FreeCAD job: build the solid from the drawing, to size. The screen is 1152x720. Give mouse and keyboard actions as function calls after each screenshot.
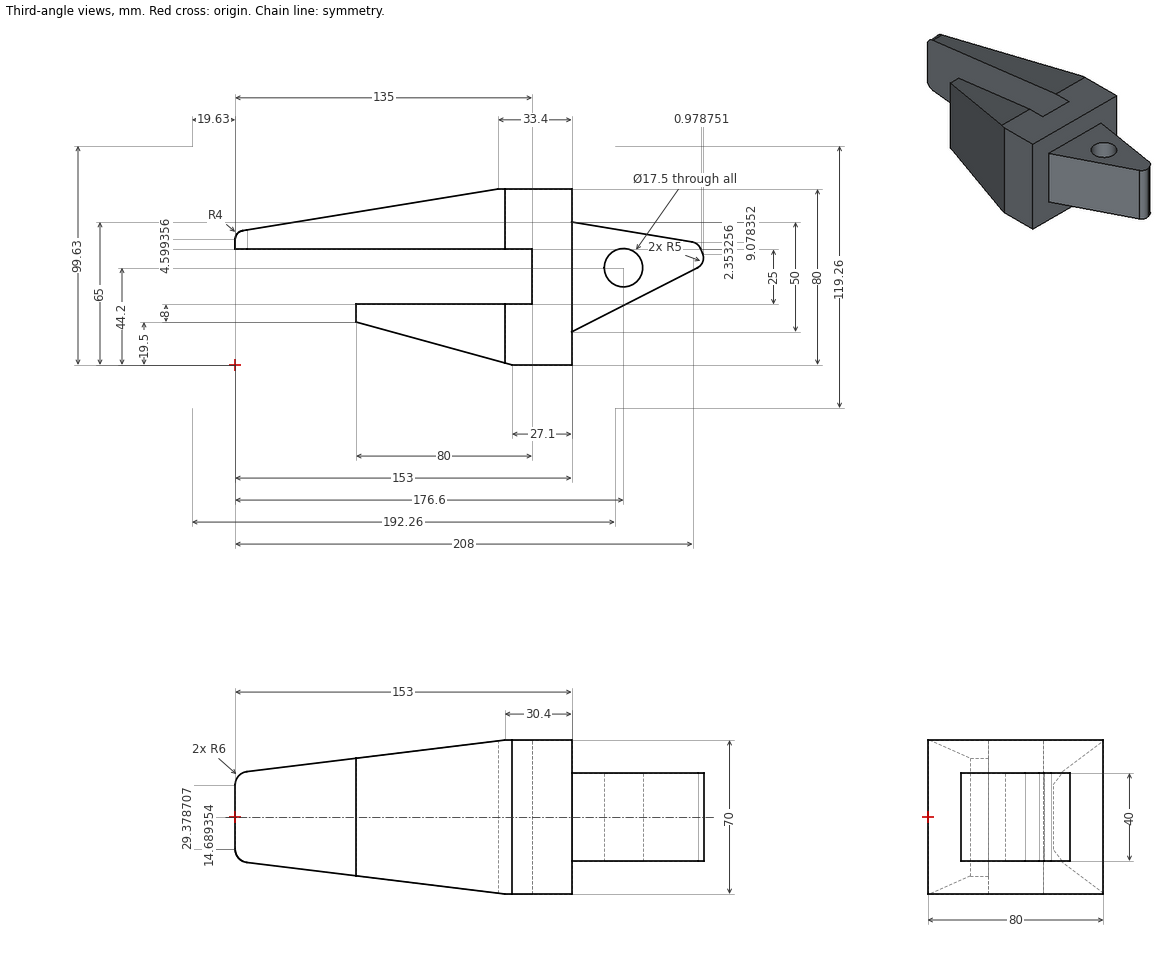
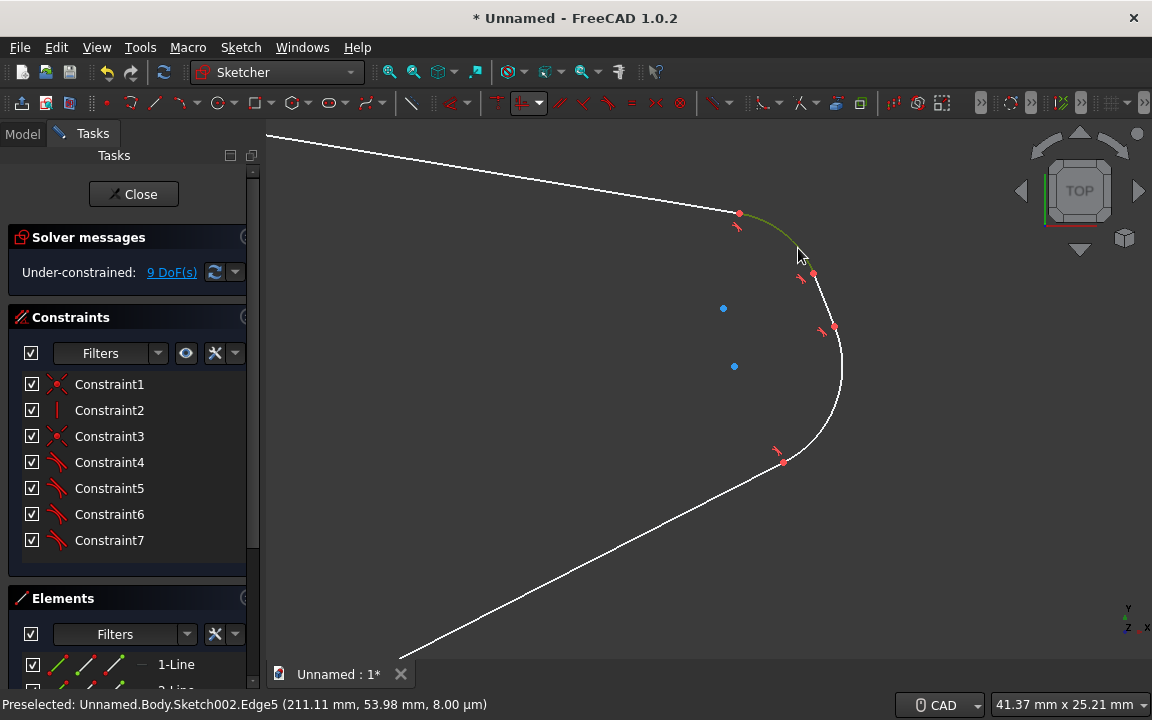
click(820, 432)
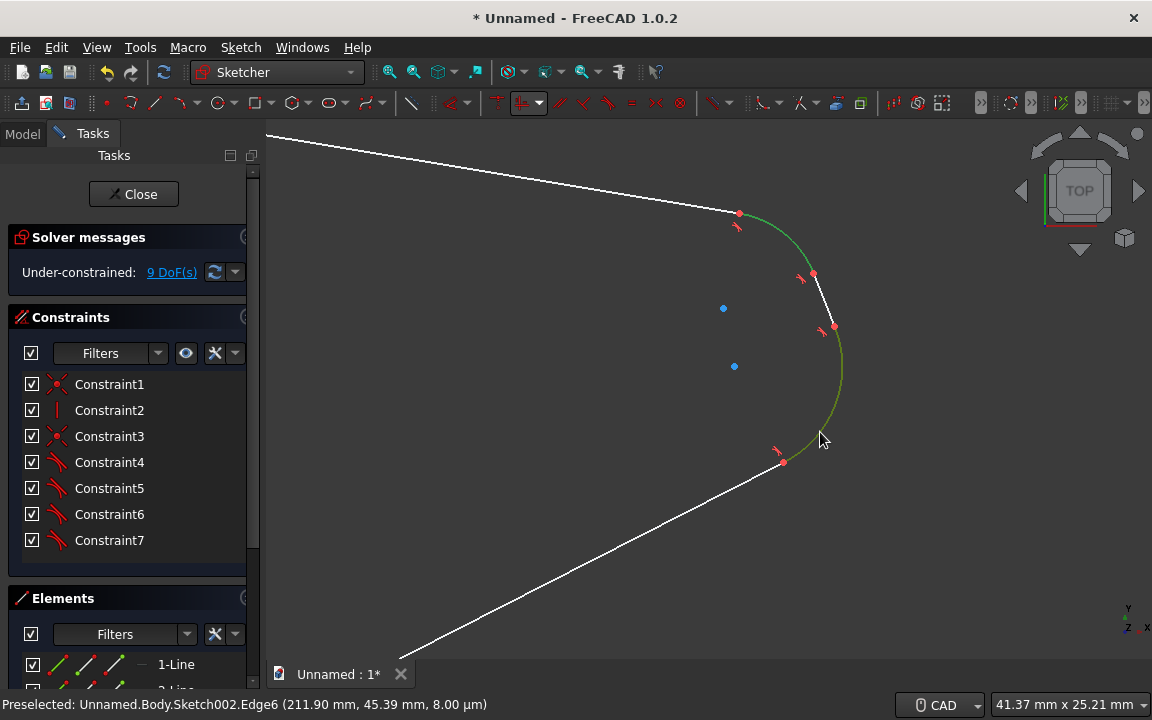
click(632, 104)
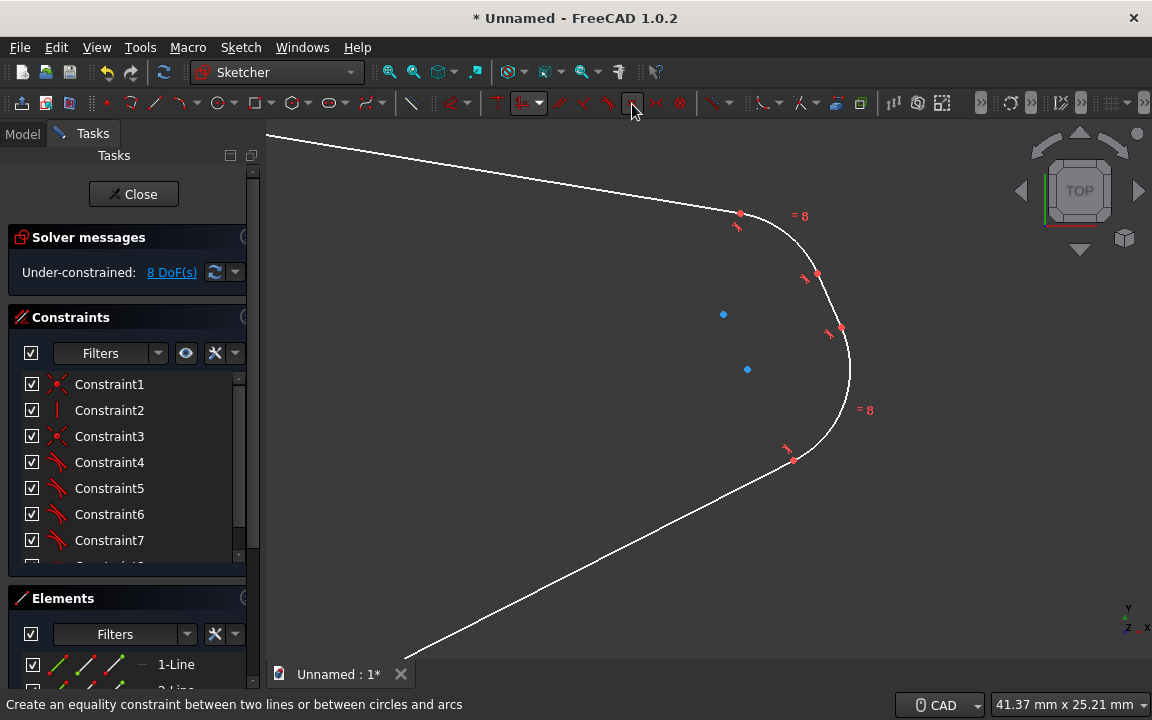
key(d)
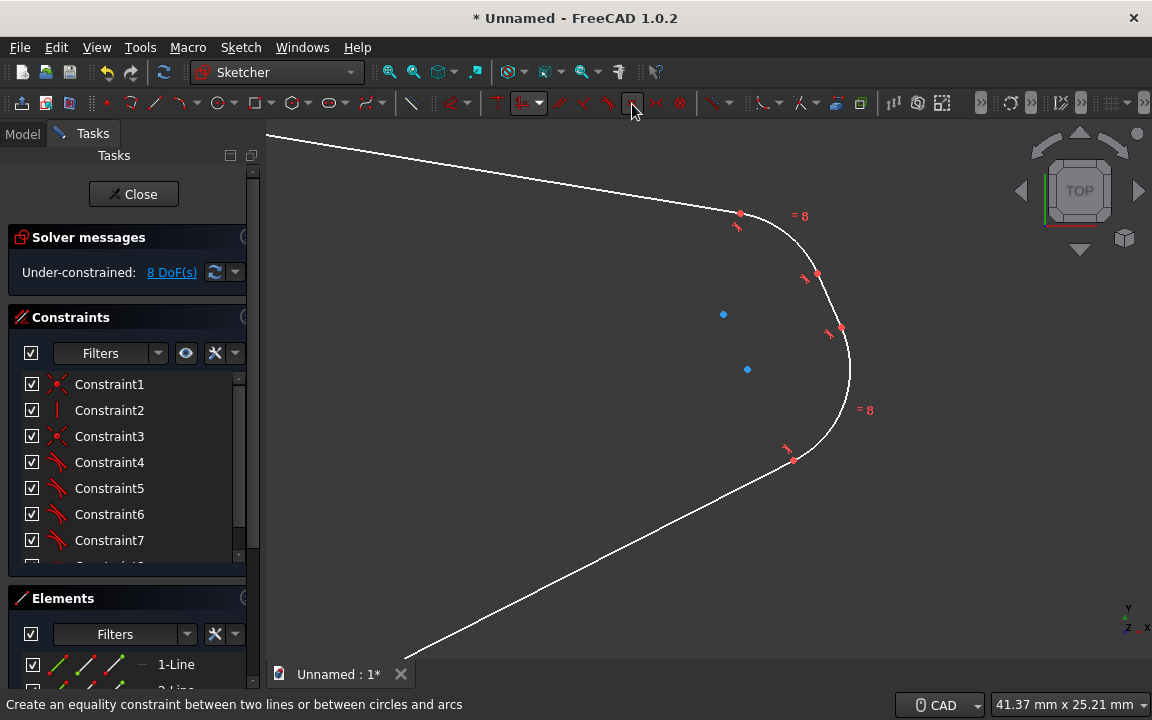
click(801, 247)
click(825, 226)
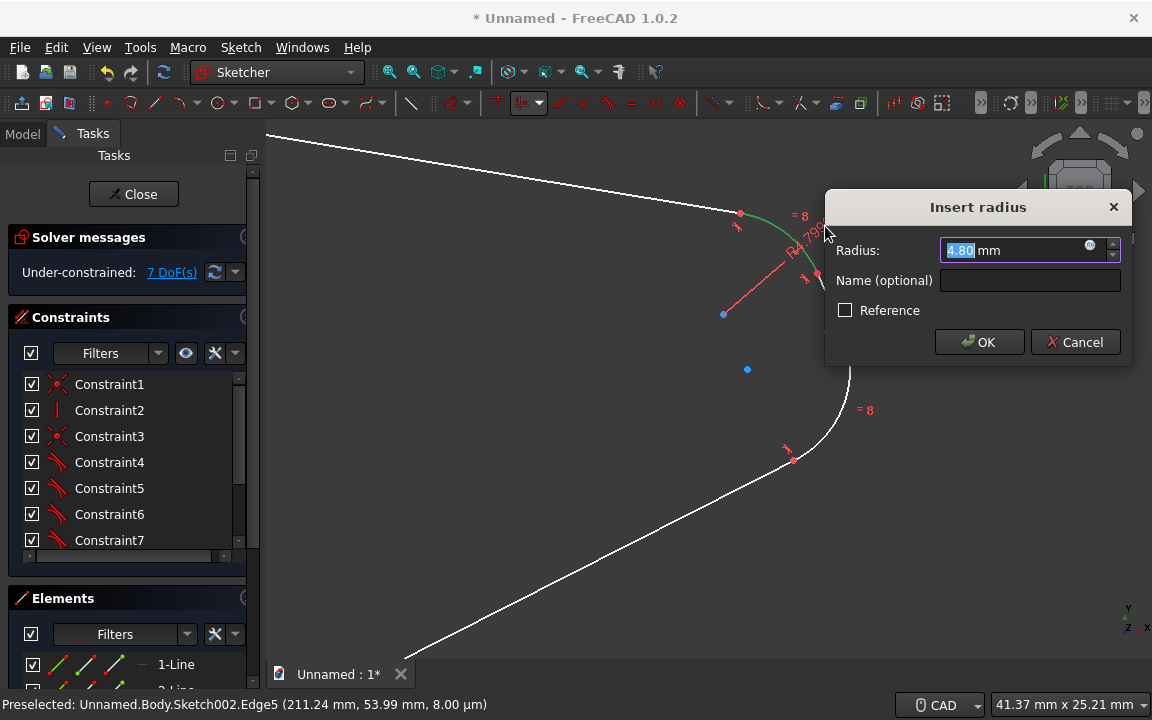
text(5)
key(Return)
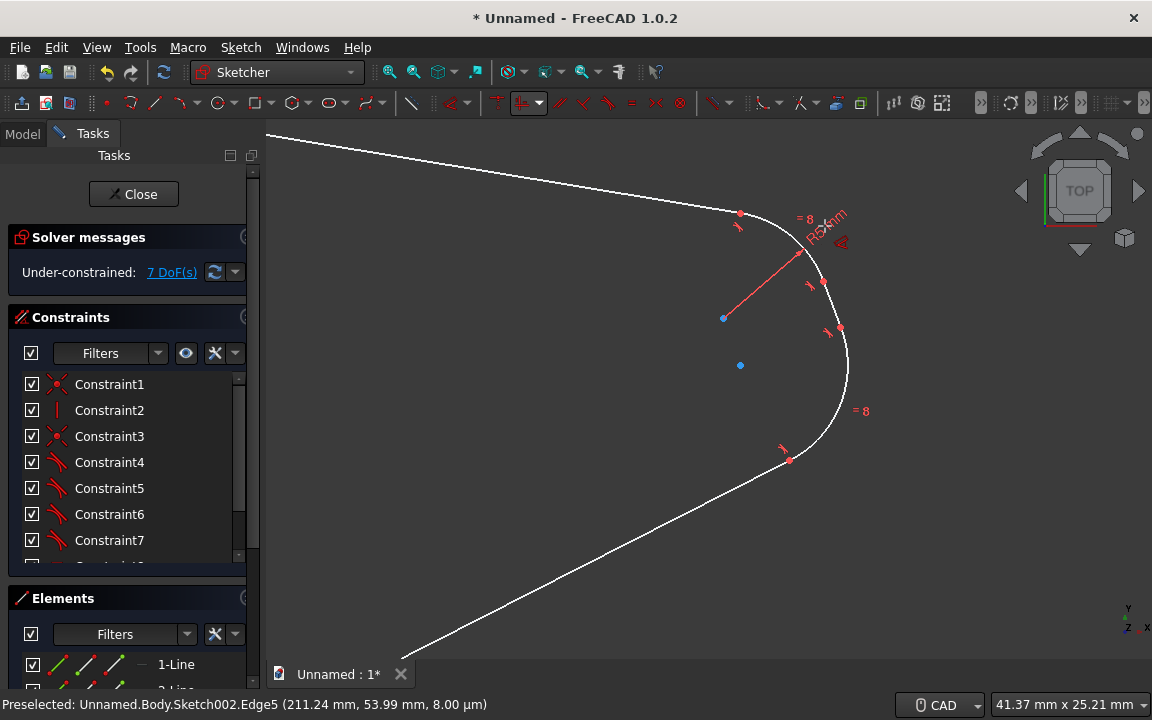
scroll(832, 319, down, 6)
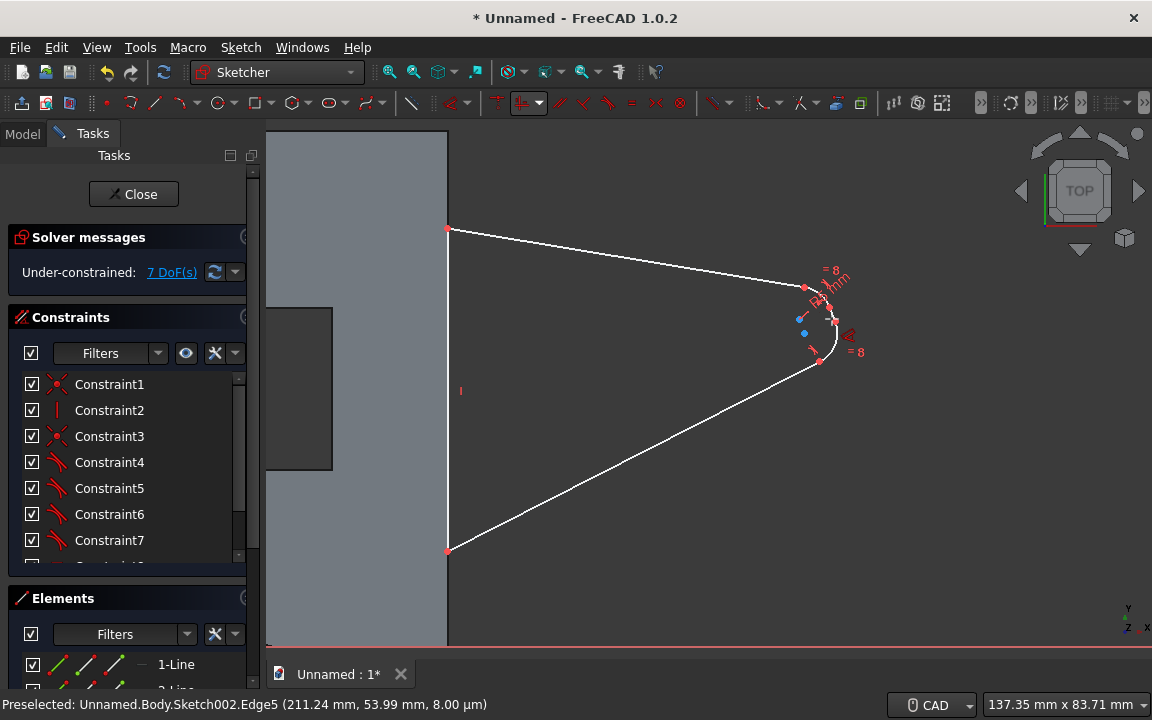
click(448, 325)
click(414, 390)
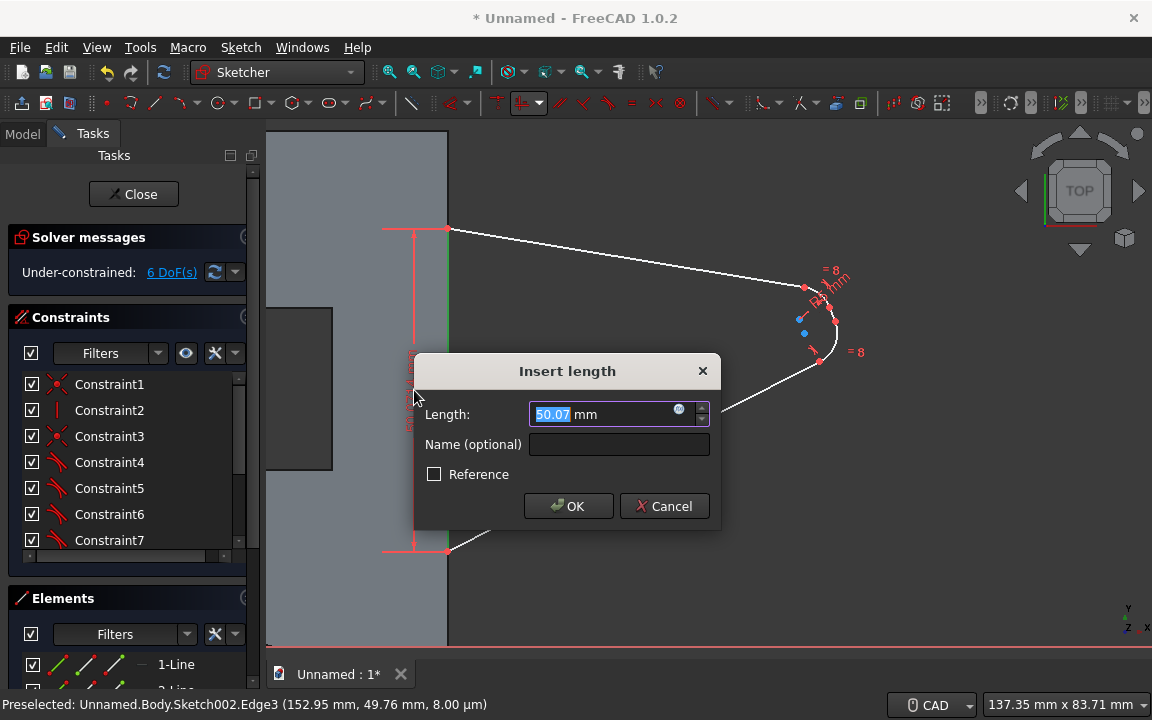
text(50)
key(Return)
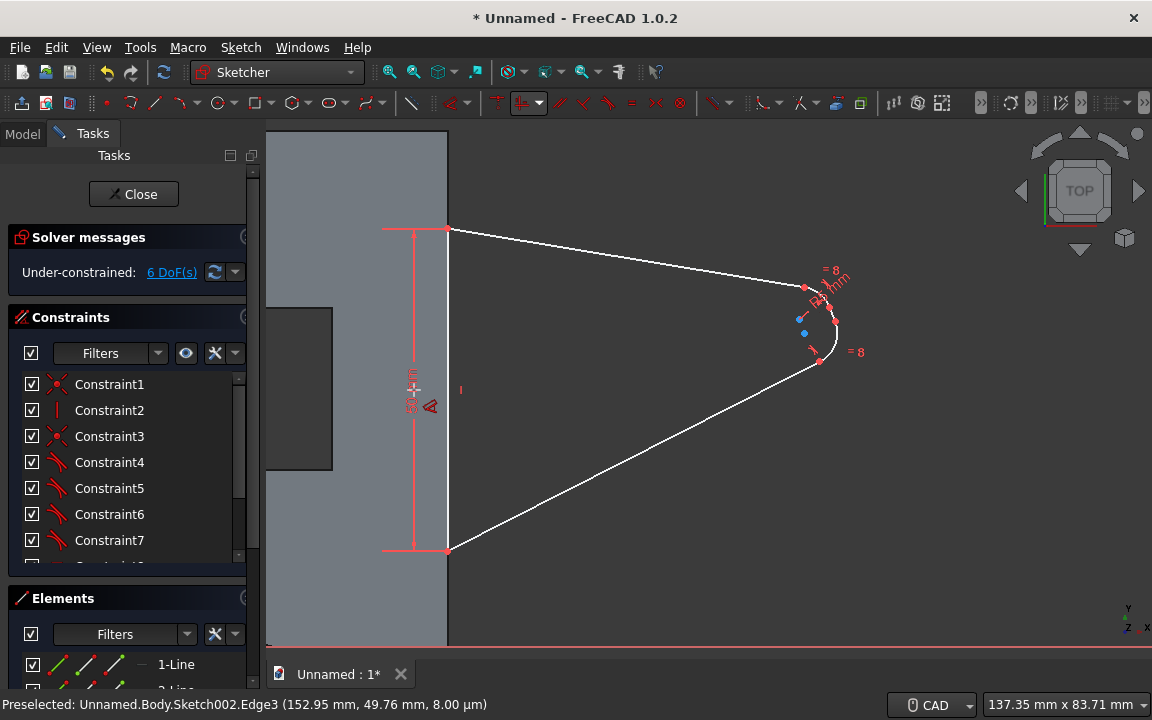
click(448, 229)
click(482, 430)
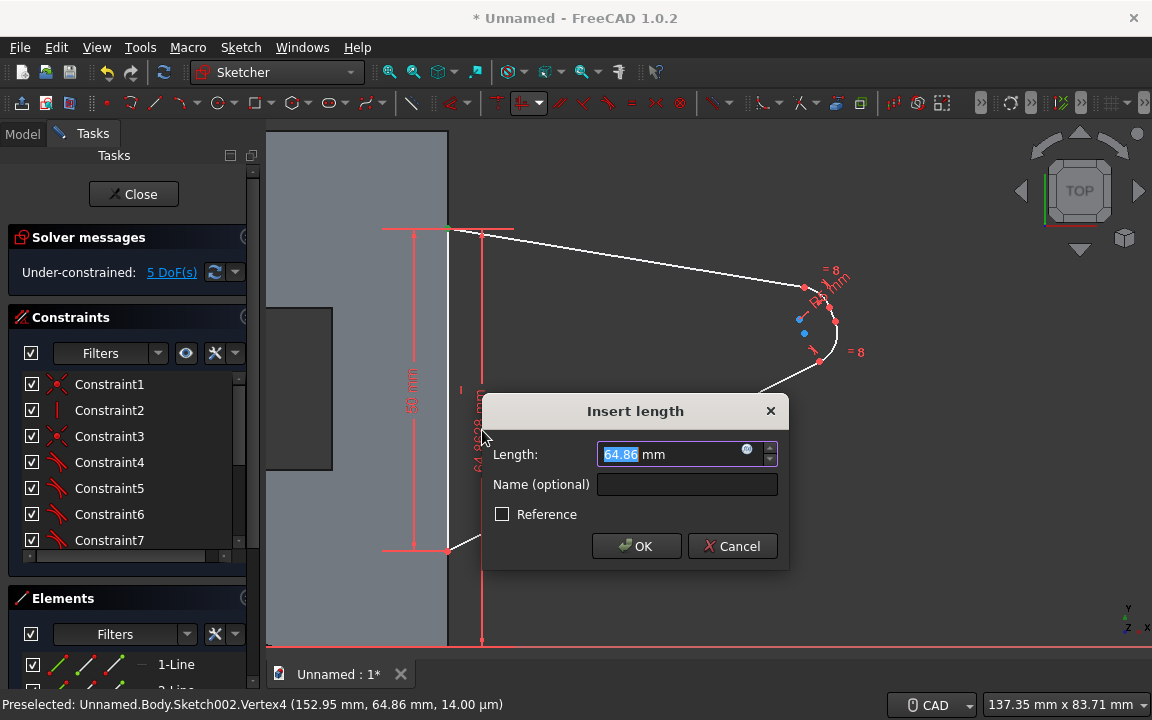
text(65)
key(Return)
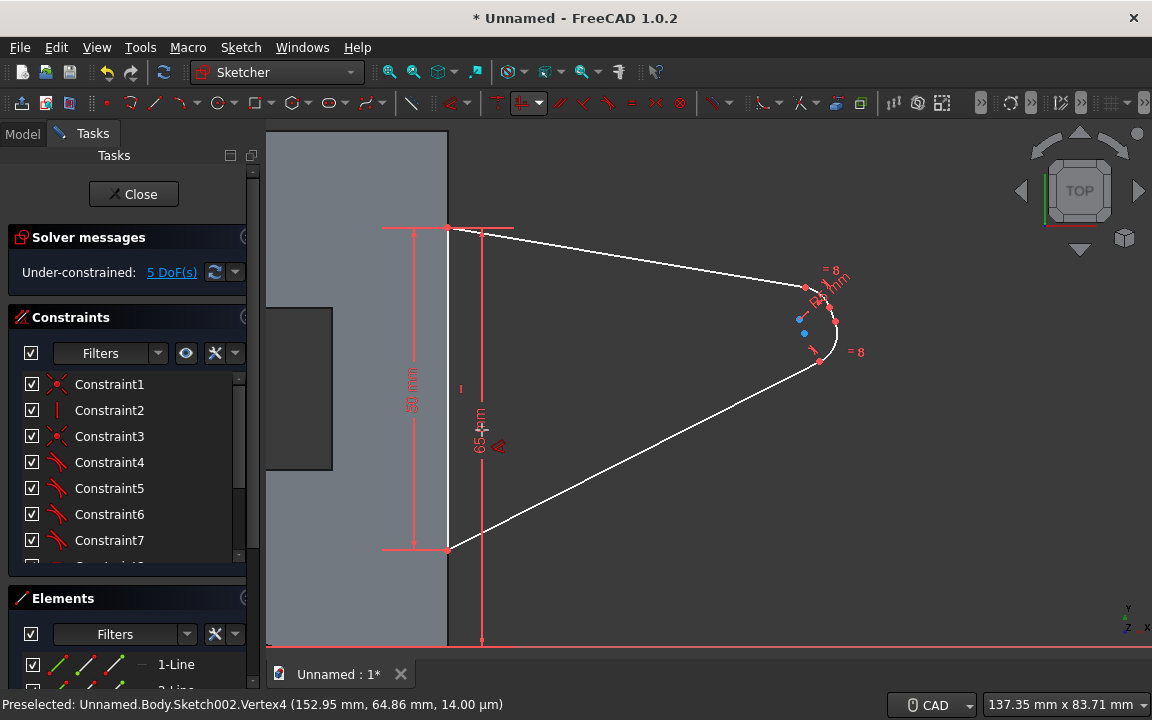
click(448, 228)
click(371, 194)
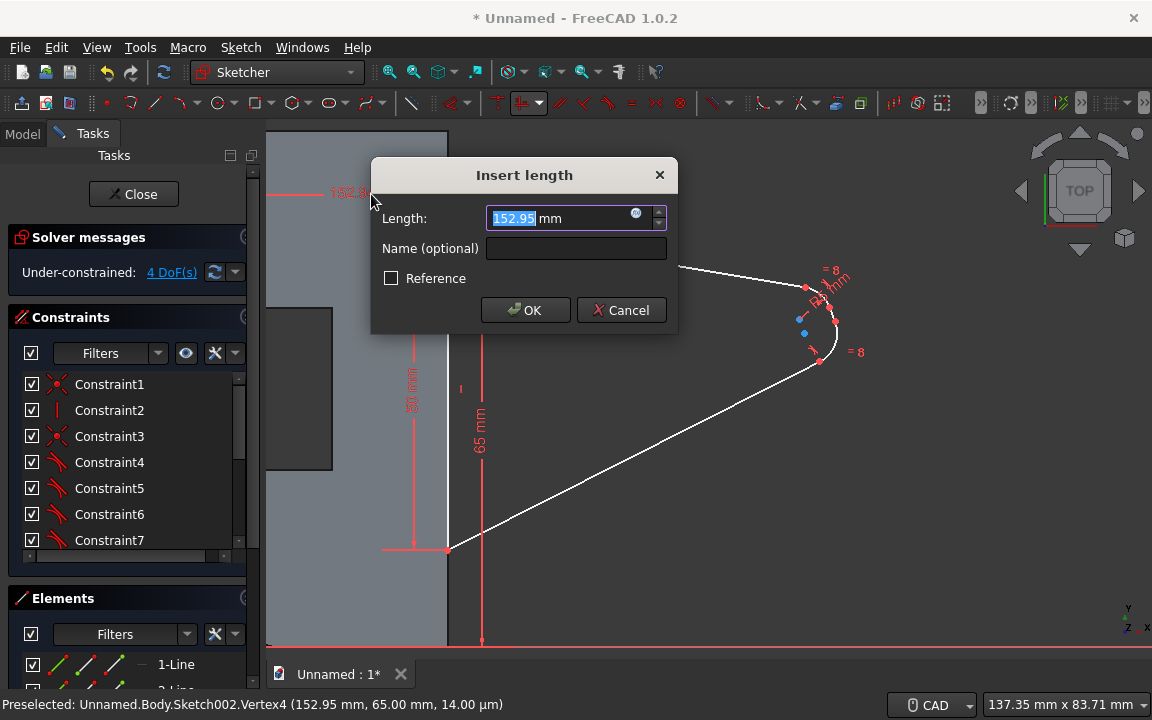
text(153)
key(Return)